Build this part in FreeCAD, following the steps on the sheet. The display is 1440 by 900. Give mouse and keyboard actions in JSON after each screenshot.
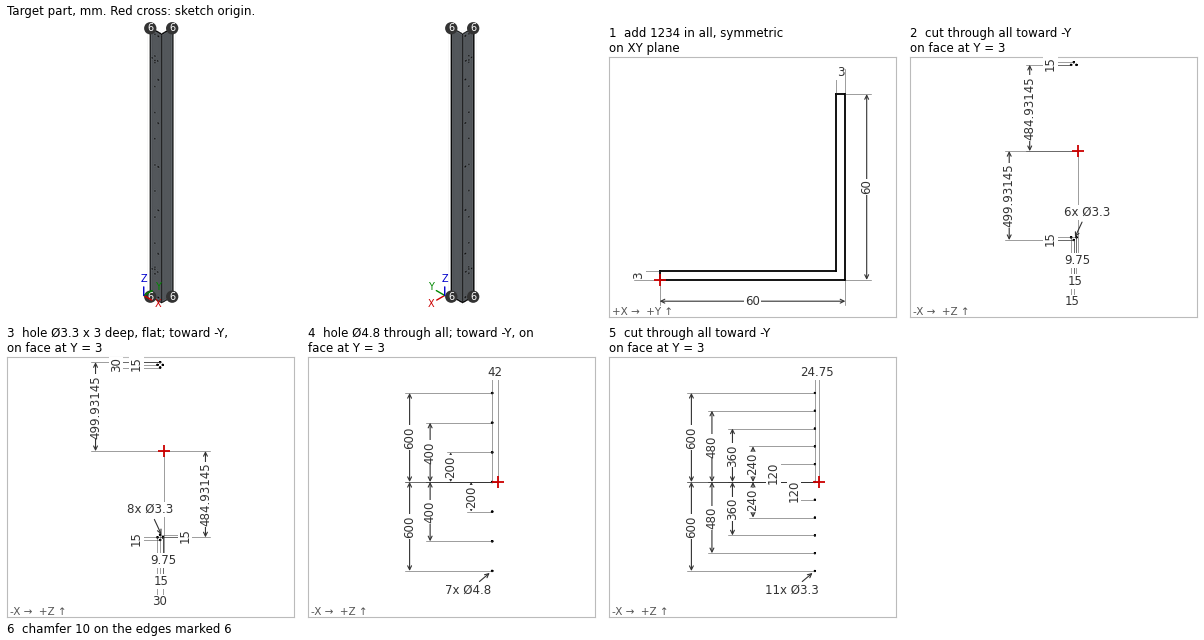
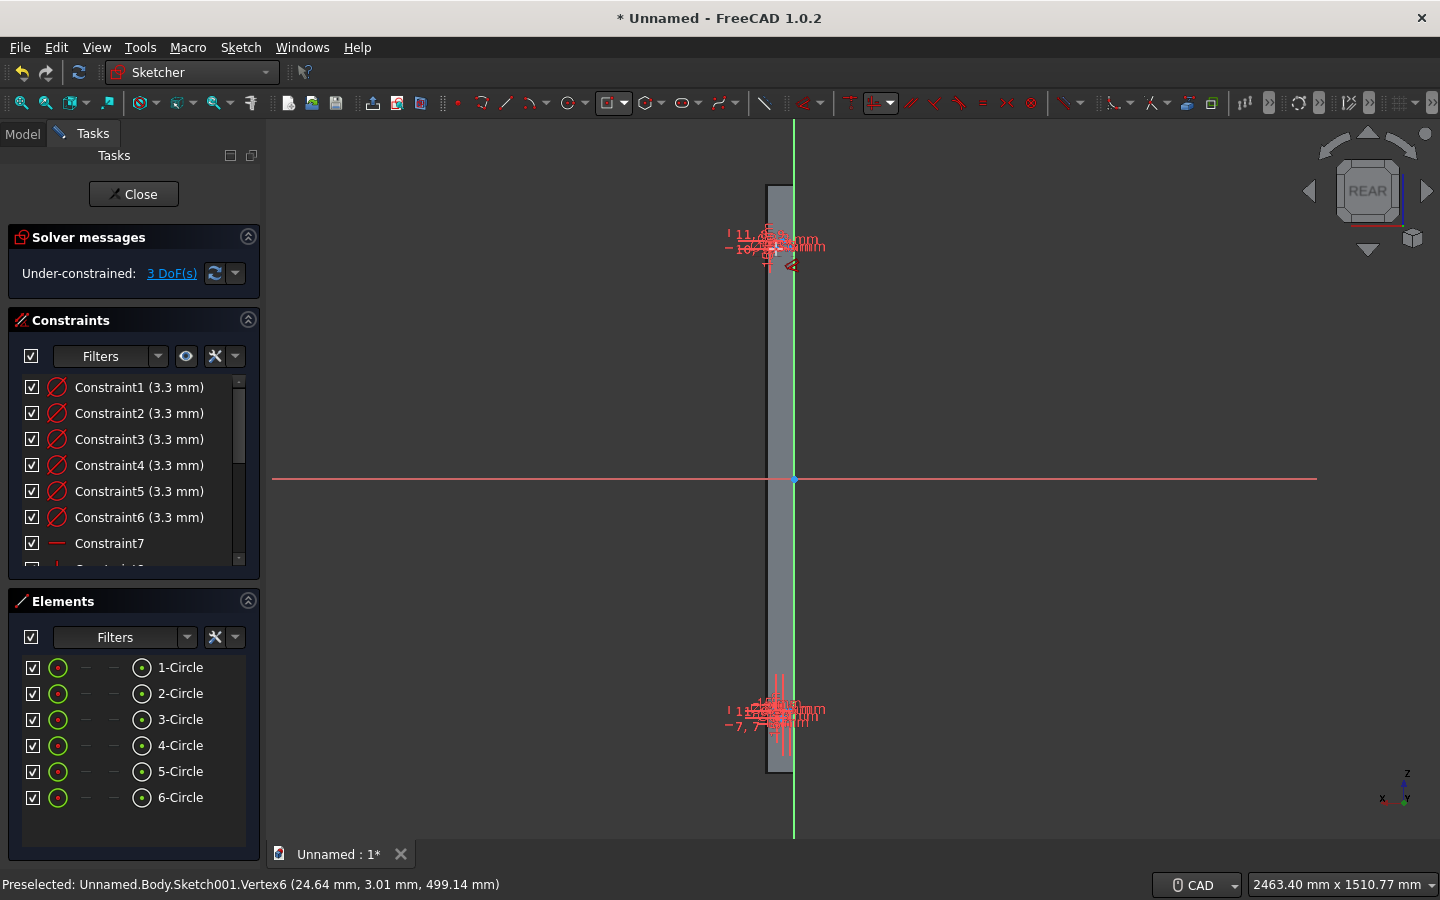
{"action": "scroll", "coordinate": [790, 711], "scroll_direction": "up", "scroll_amount": 11}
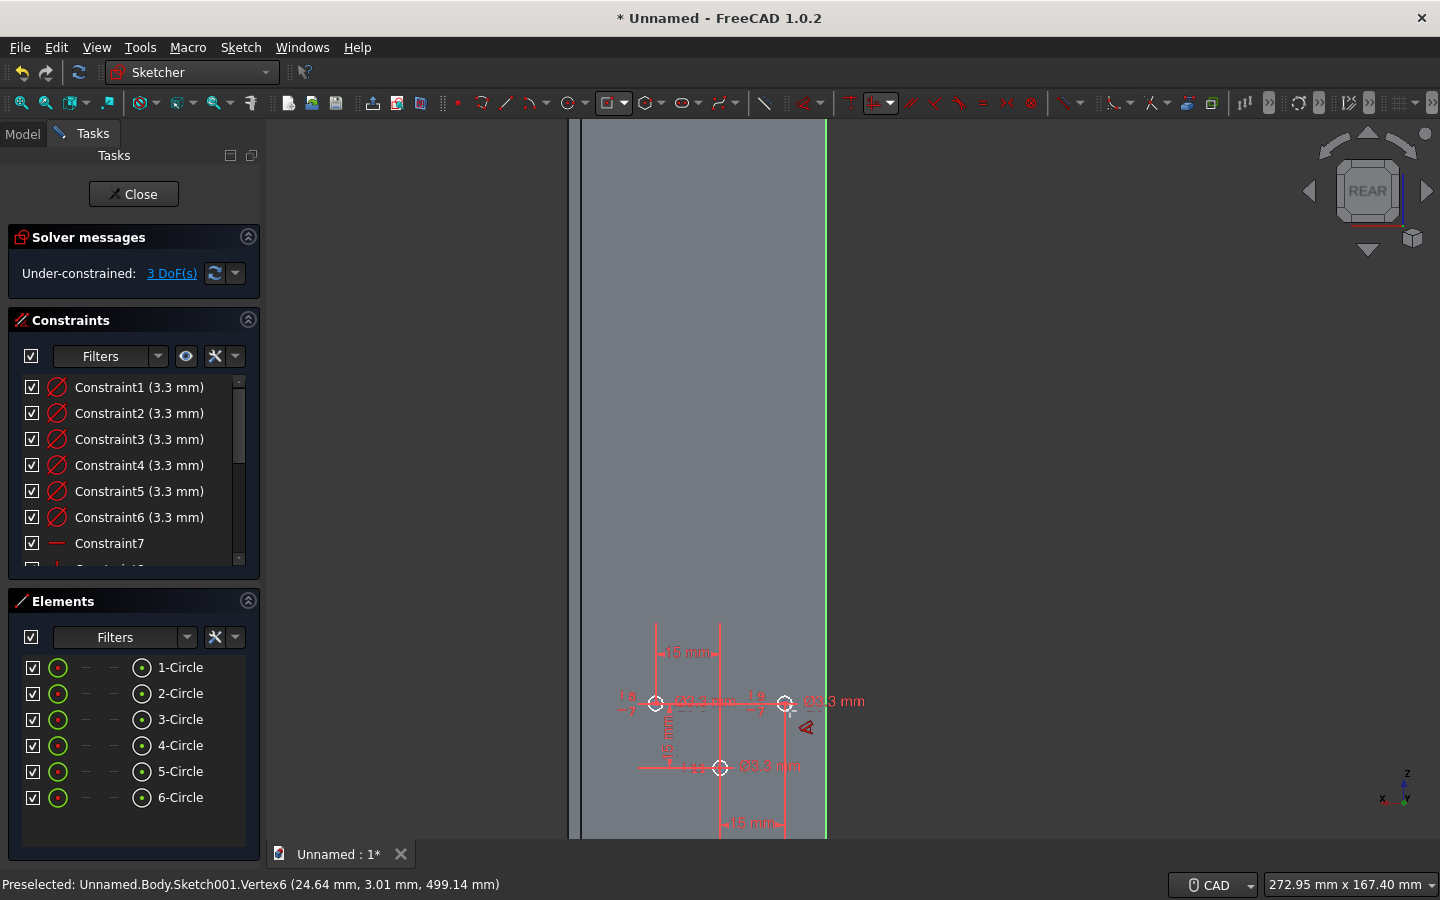
{"action": "left_click", "coordinate": [785, 704]}
{"action": "left_click", "coordinate": [805, 738]}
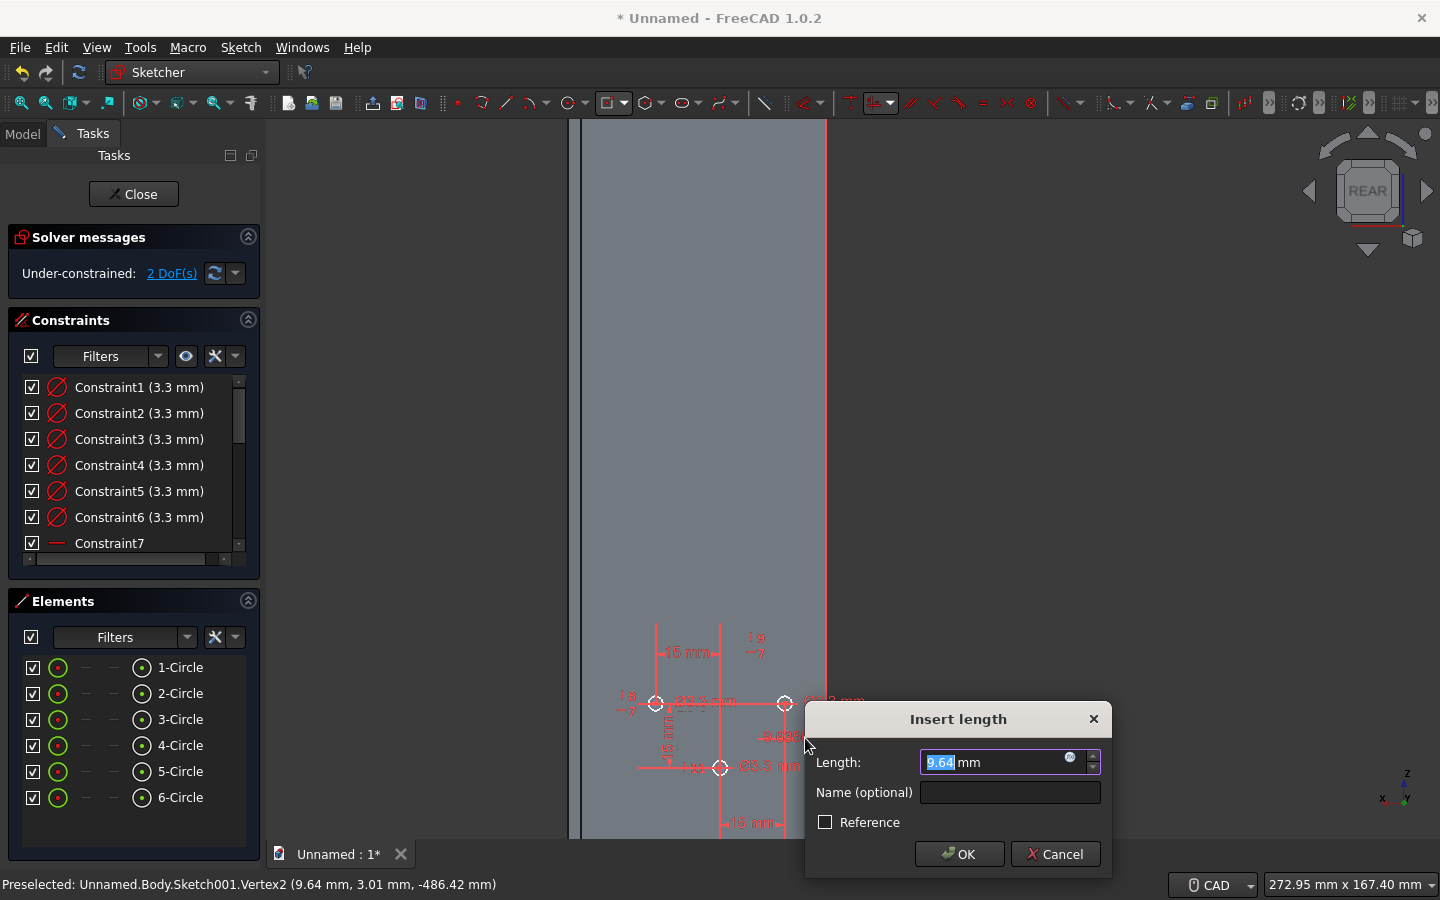
{"action": "type", "text": "9.75"}
{"action": "key", "text": "Return"}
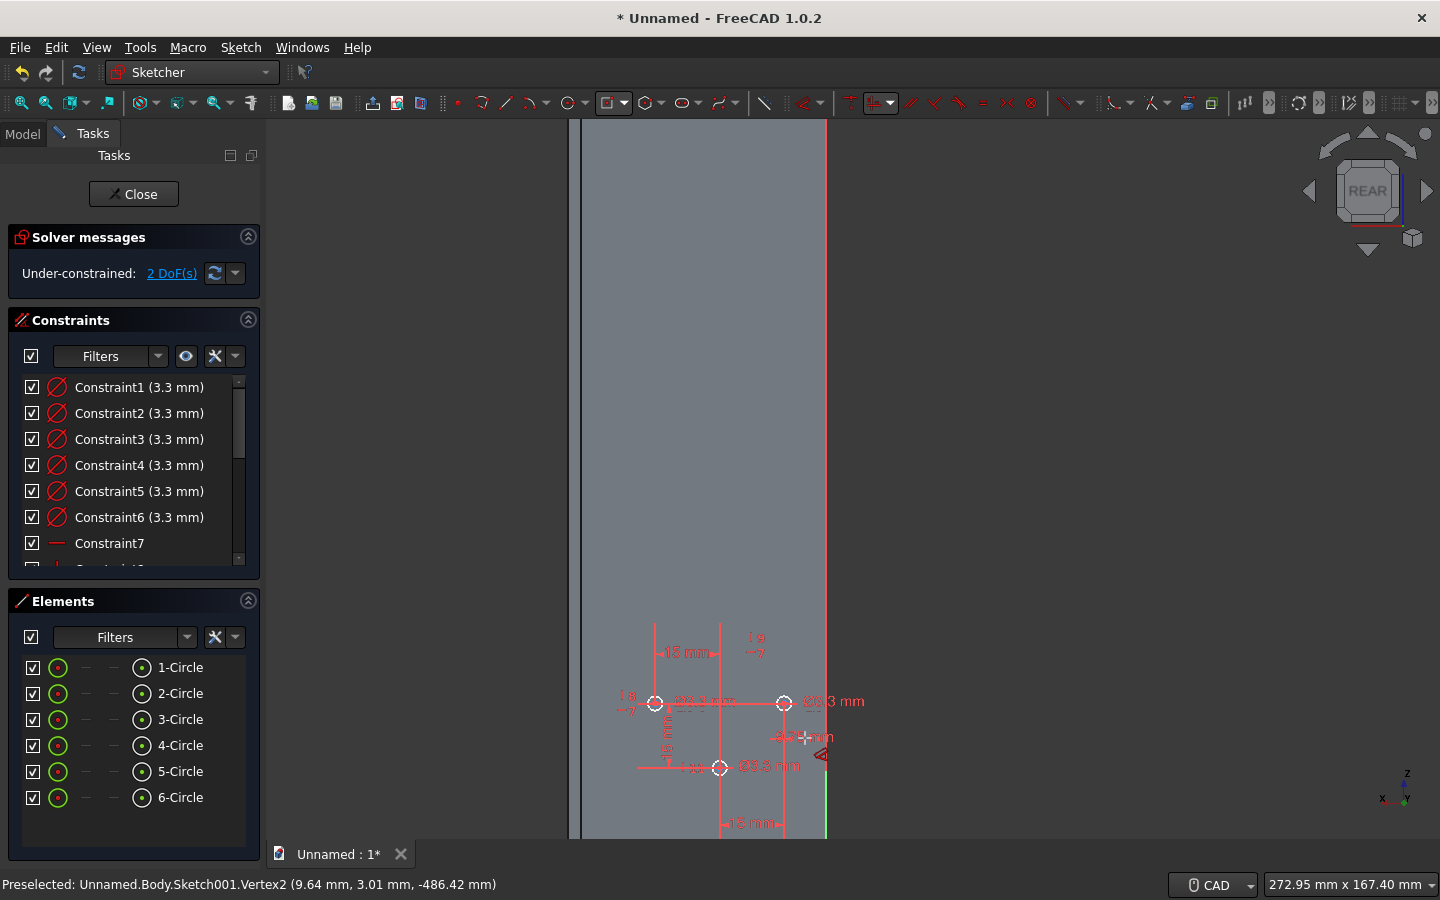
{"action": "scroll", "coordinate": [790, 712], "scroll_direction": "down", "scroll_amount": 11}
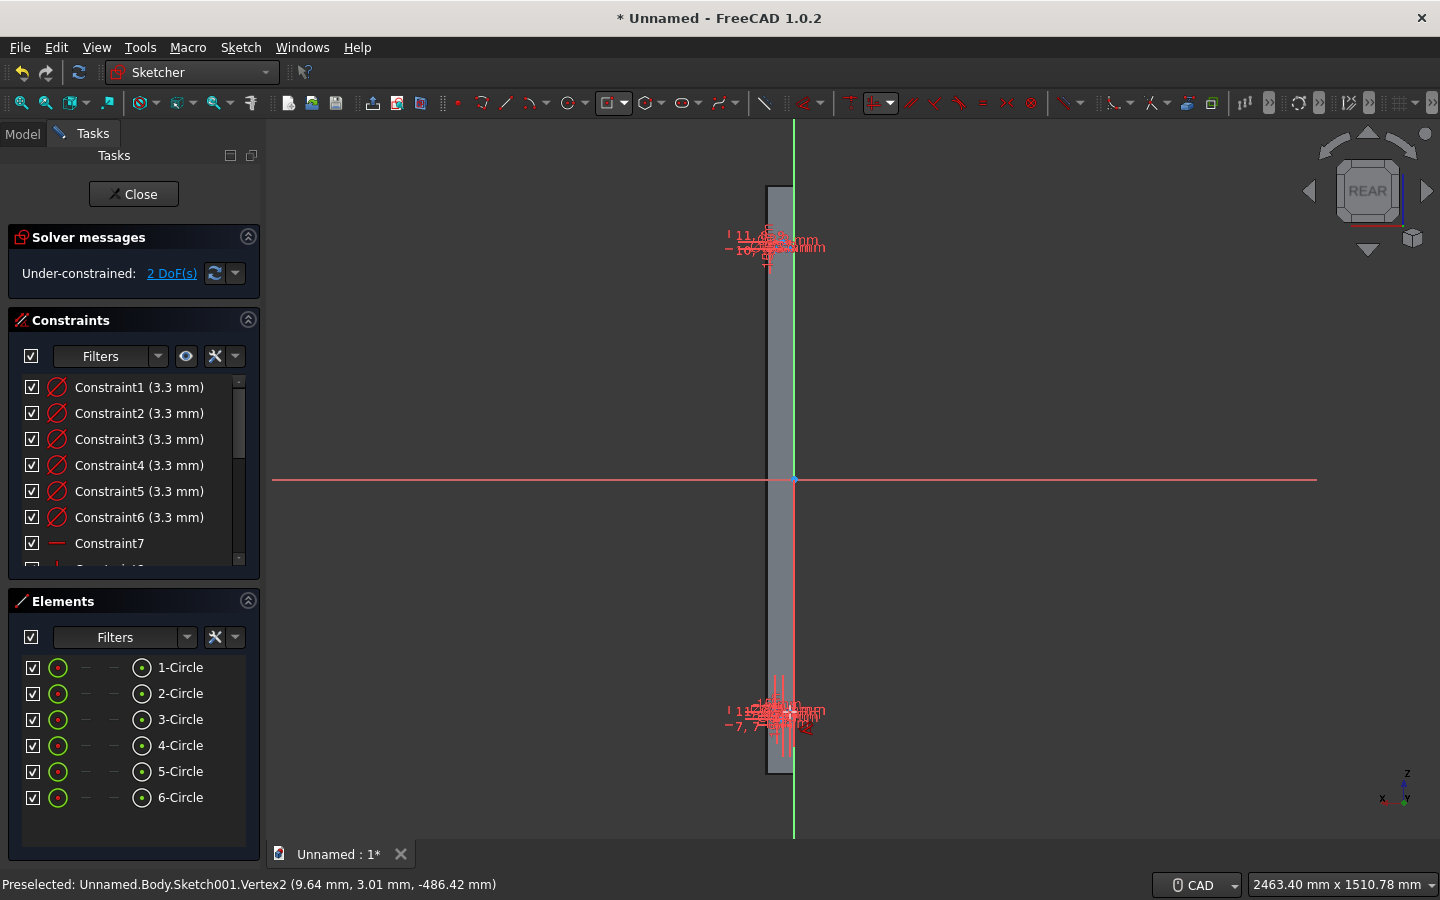
{"action": "left_click", "coordinate": [783, 719]}
{"action": "left_click", "coordinate": [828, 599]}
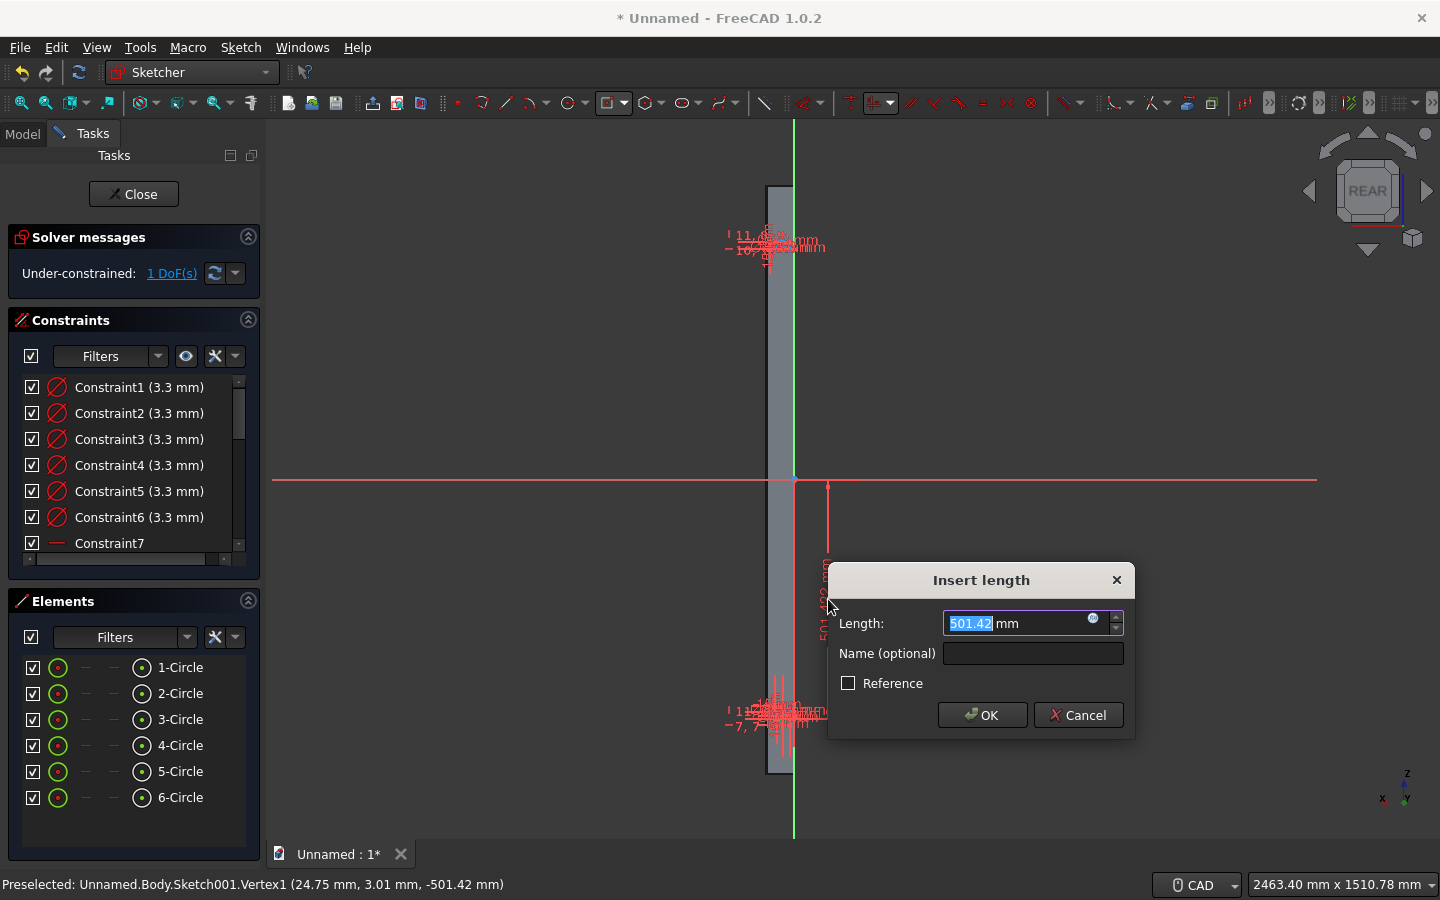
{"action": "type", "text": "499.93145"}
{"action": "key", "text": "Return"}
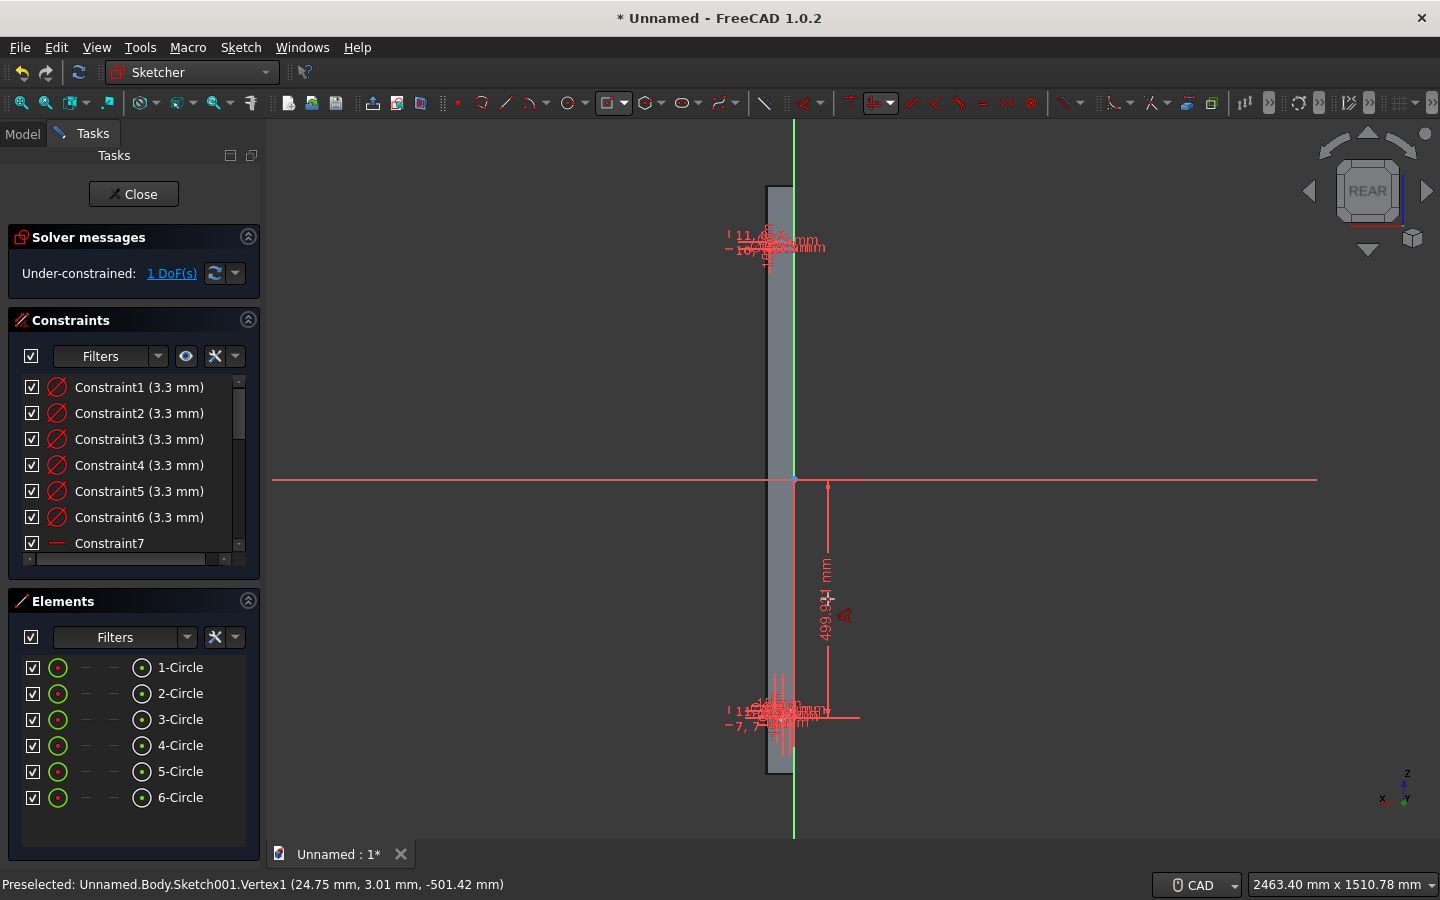
{"action": "left_click", "coordinate": [775, 249]}
{"action": "left_click", "coordinate": [828, 365]}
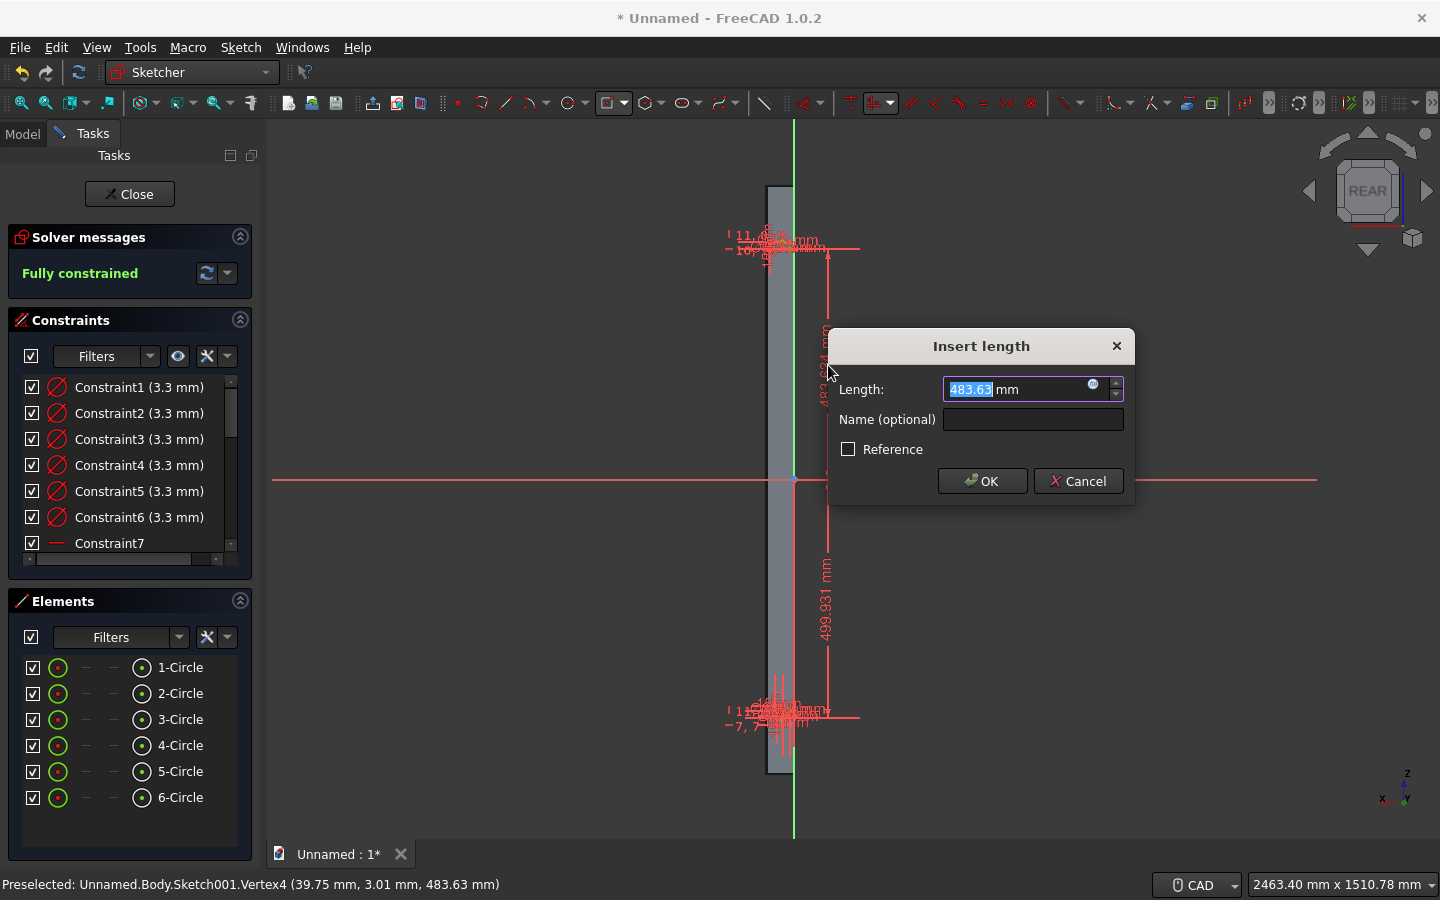
{"action": "type", "text": "484.93145"}
{"action": "key", "text": "Return"}
{"action": "key", "text": "Escape"}